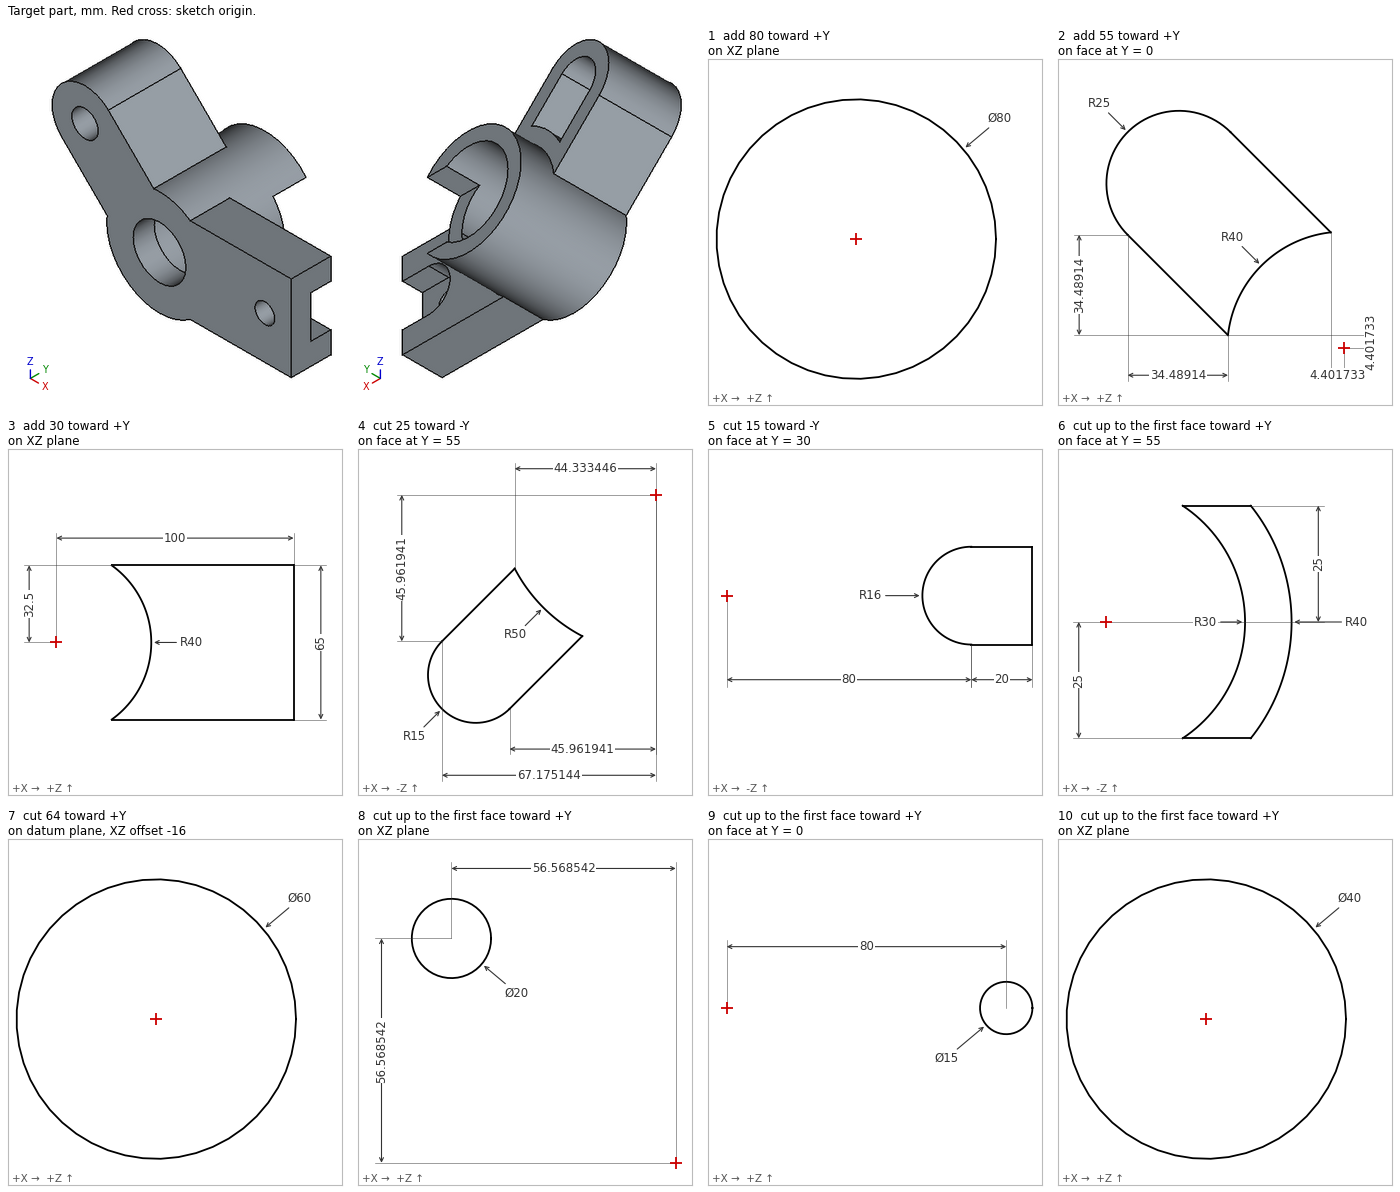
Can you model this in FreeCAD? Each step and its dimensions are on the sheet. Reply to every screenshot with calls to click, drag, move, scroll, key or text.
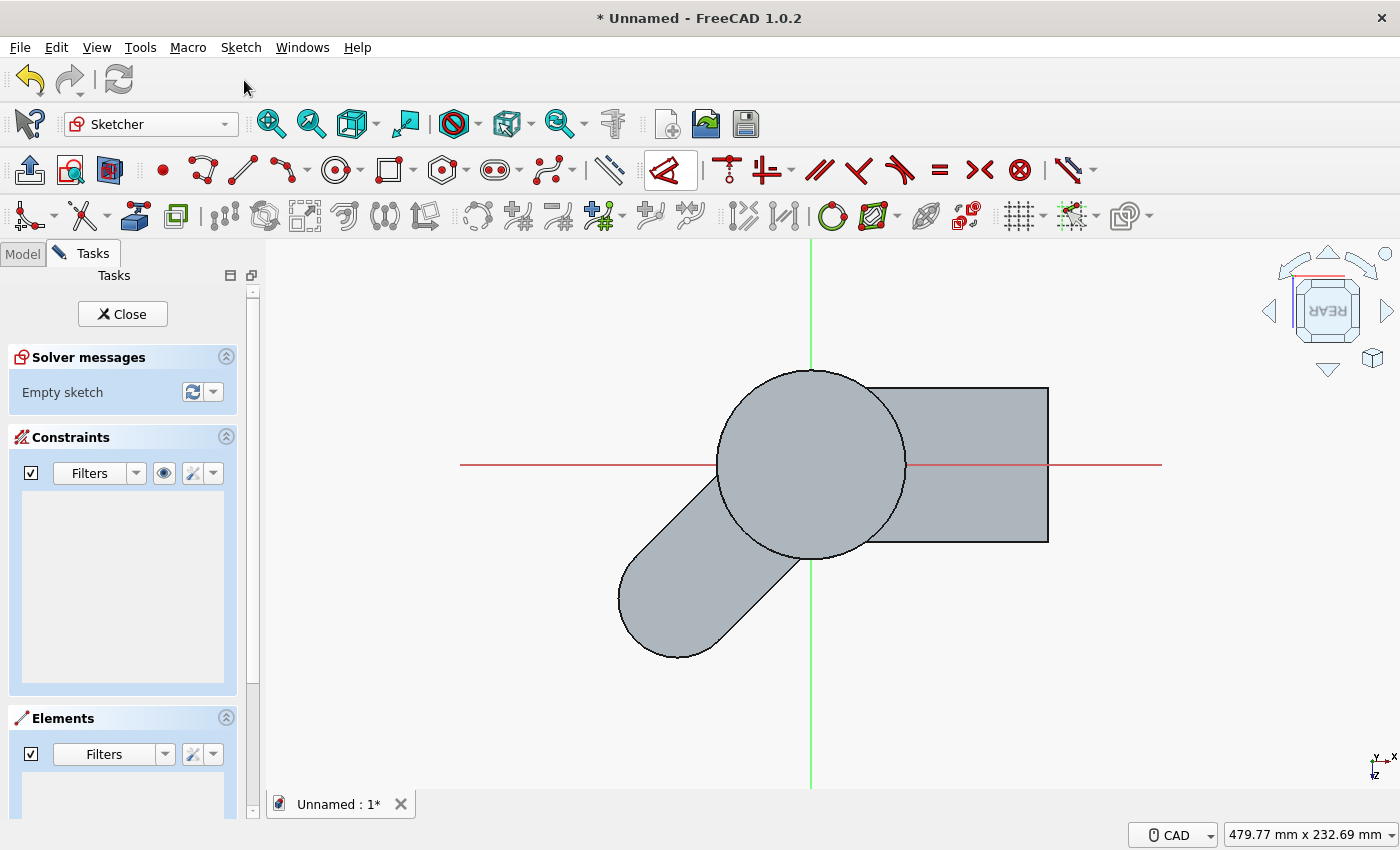
scroll(705, 569, up, 4)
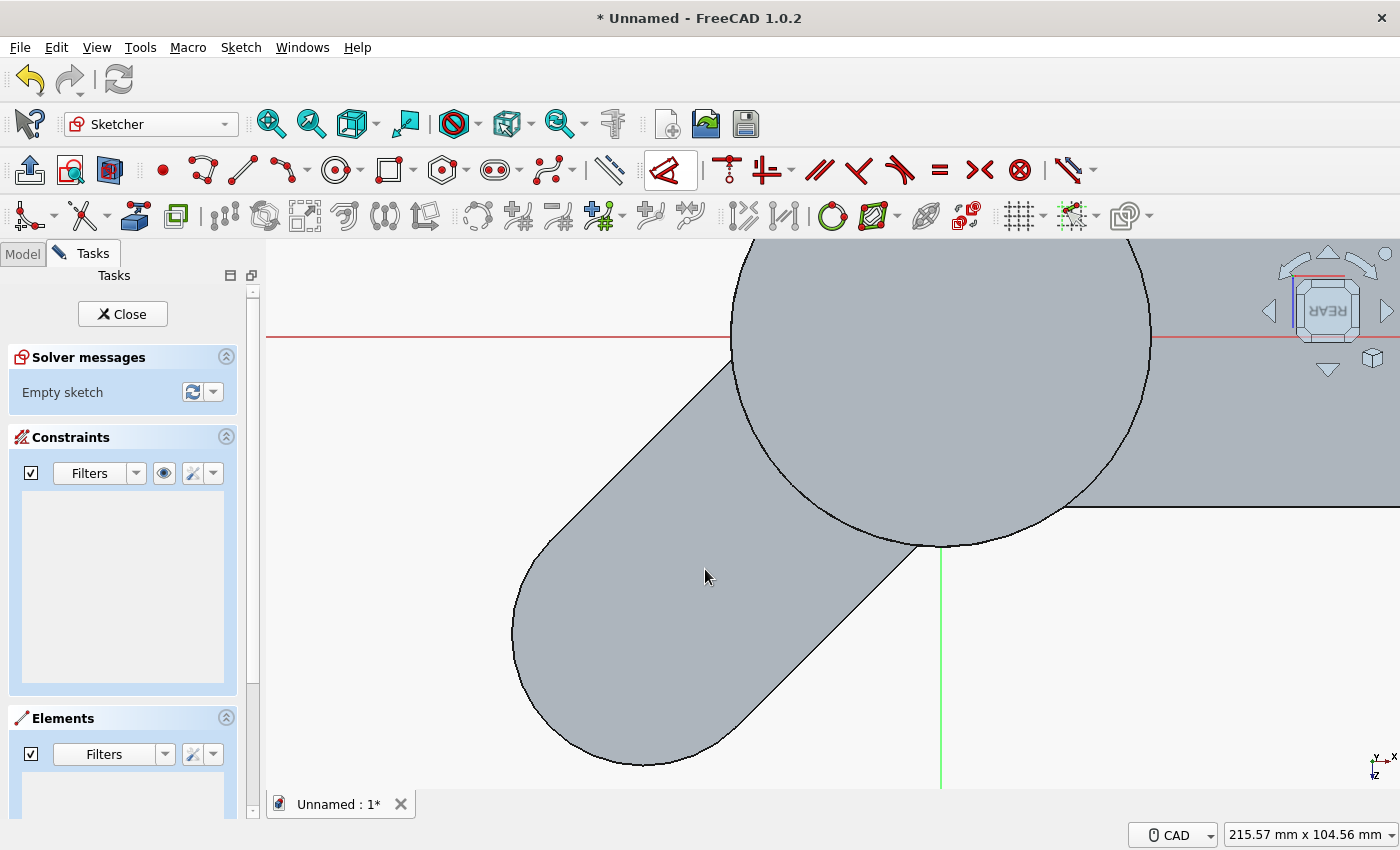
click(244, 170)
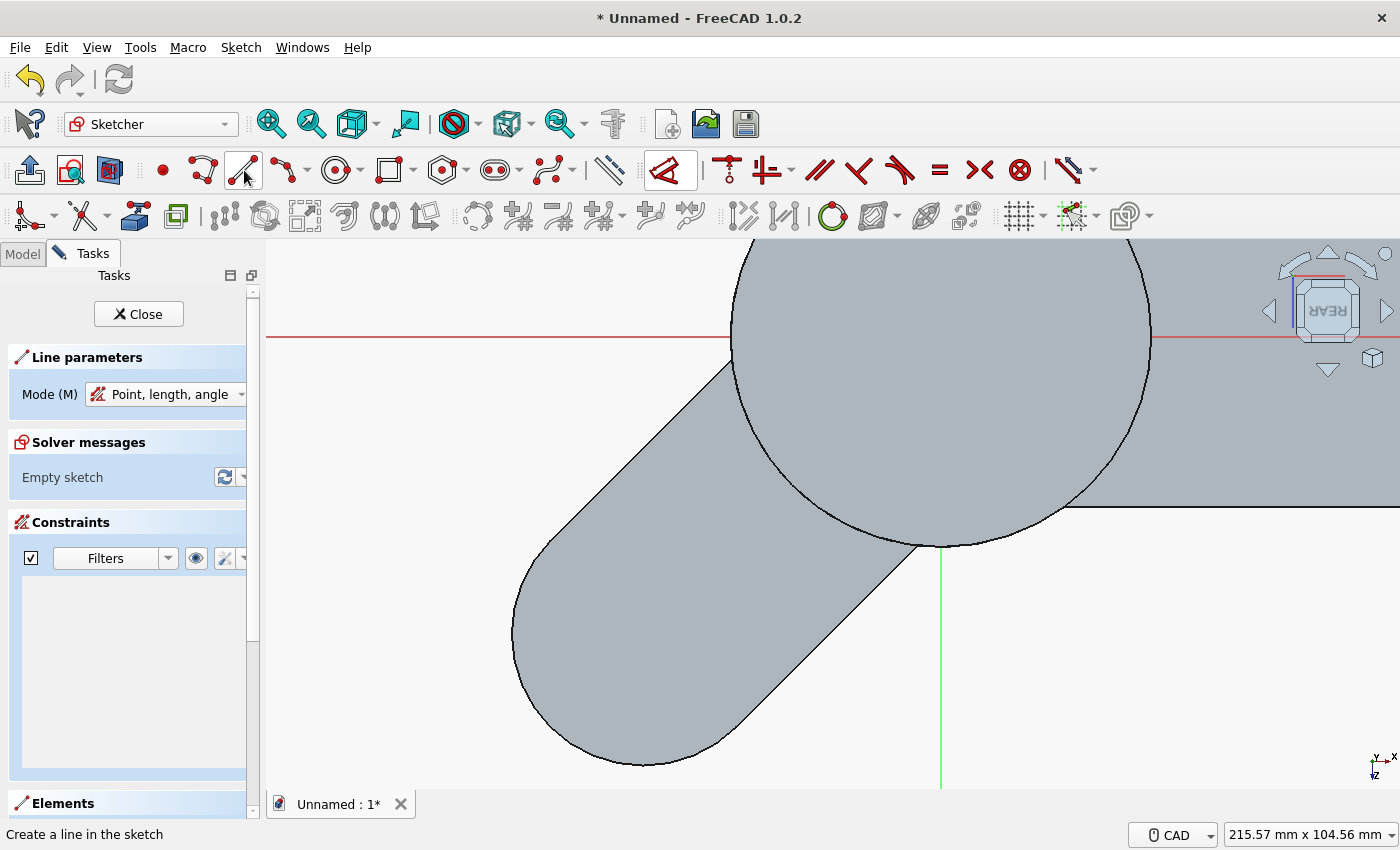
click(708, 458)
click(588, 578)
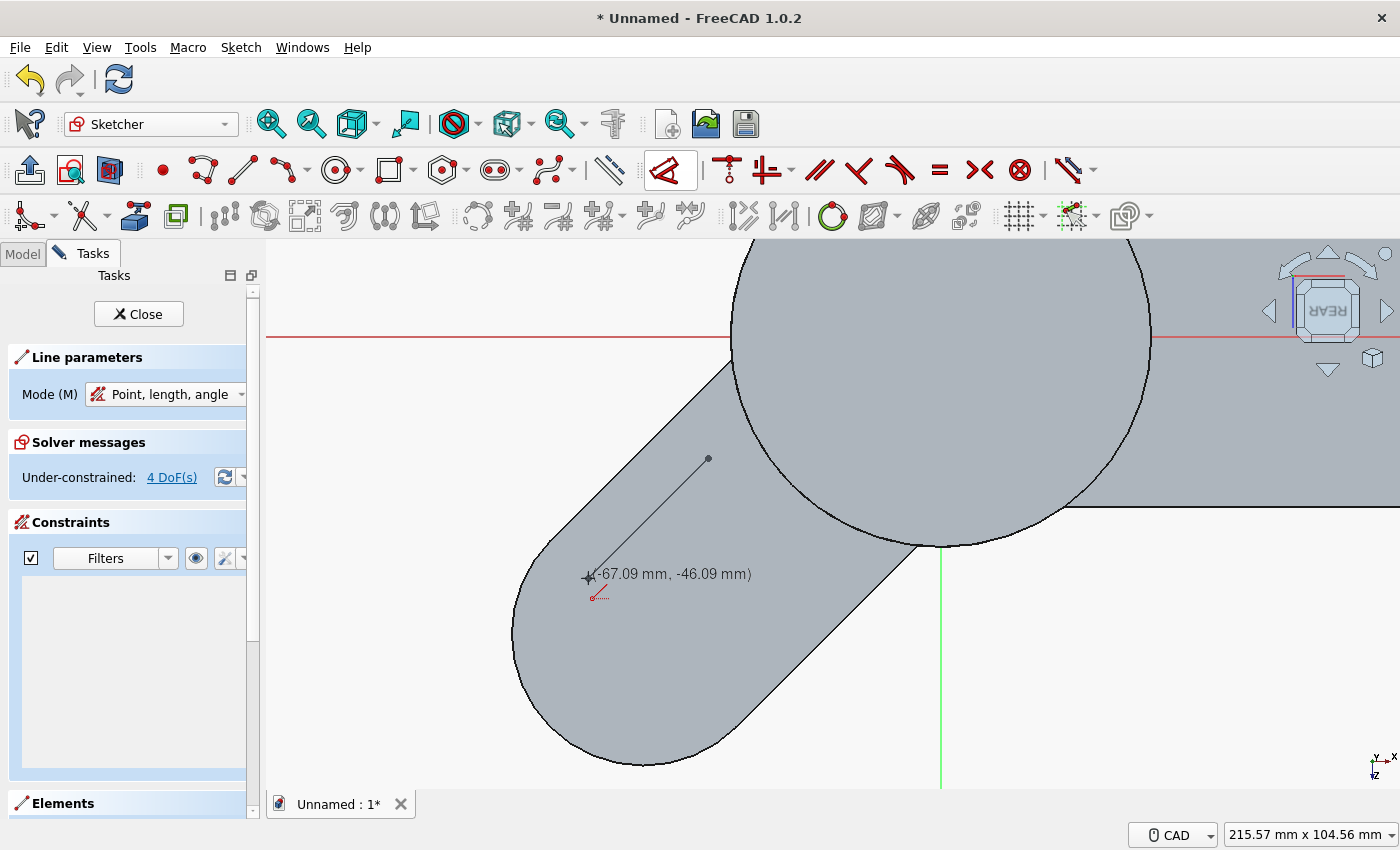
click(699, 690)
click(819, 570)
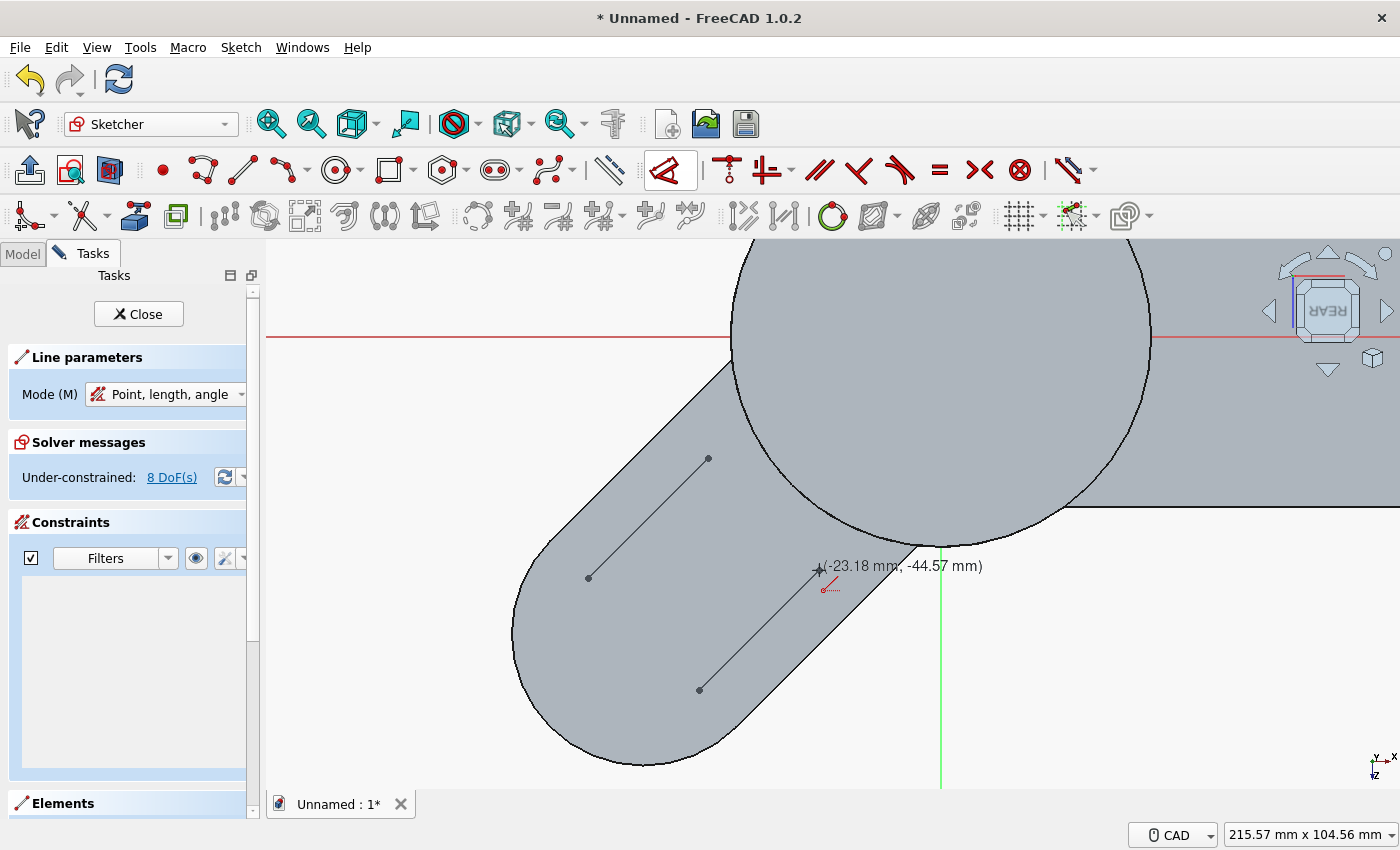
click(284, 170)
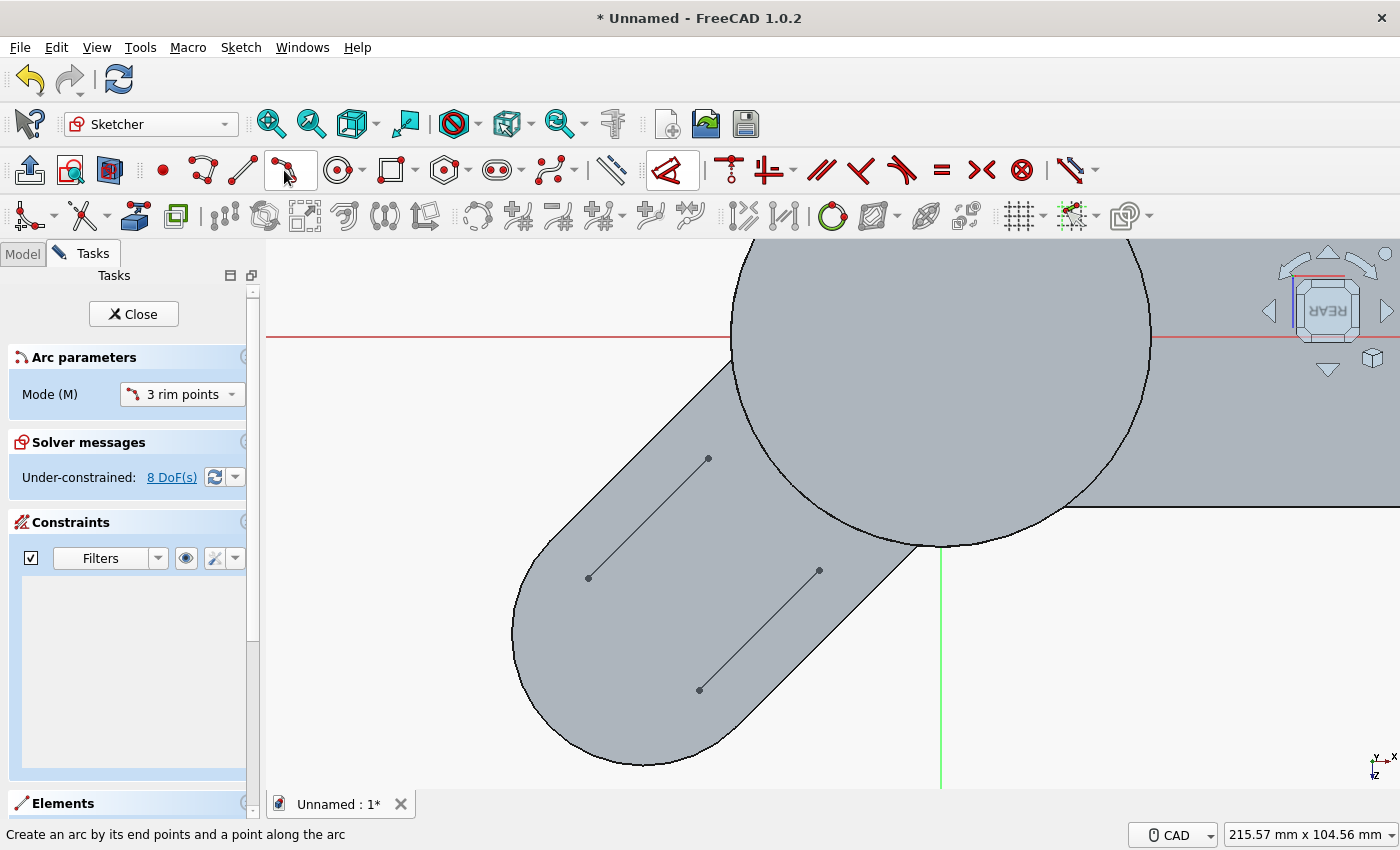
click(588, 579)
click(699, 691)
click(588, 690)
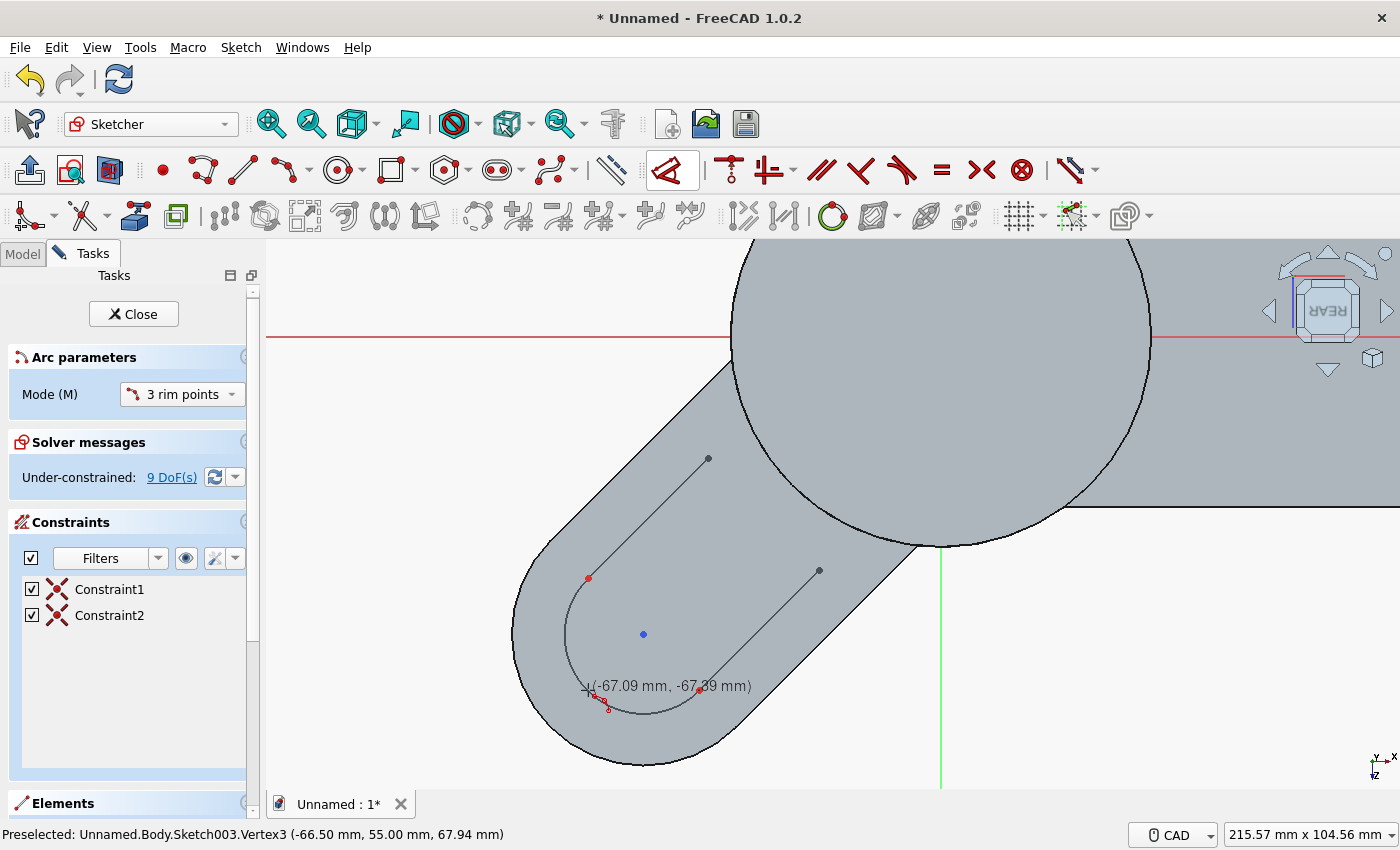
click(819, 571)
click(708, 459)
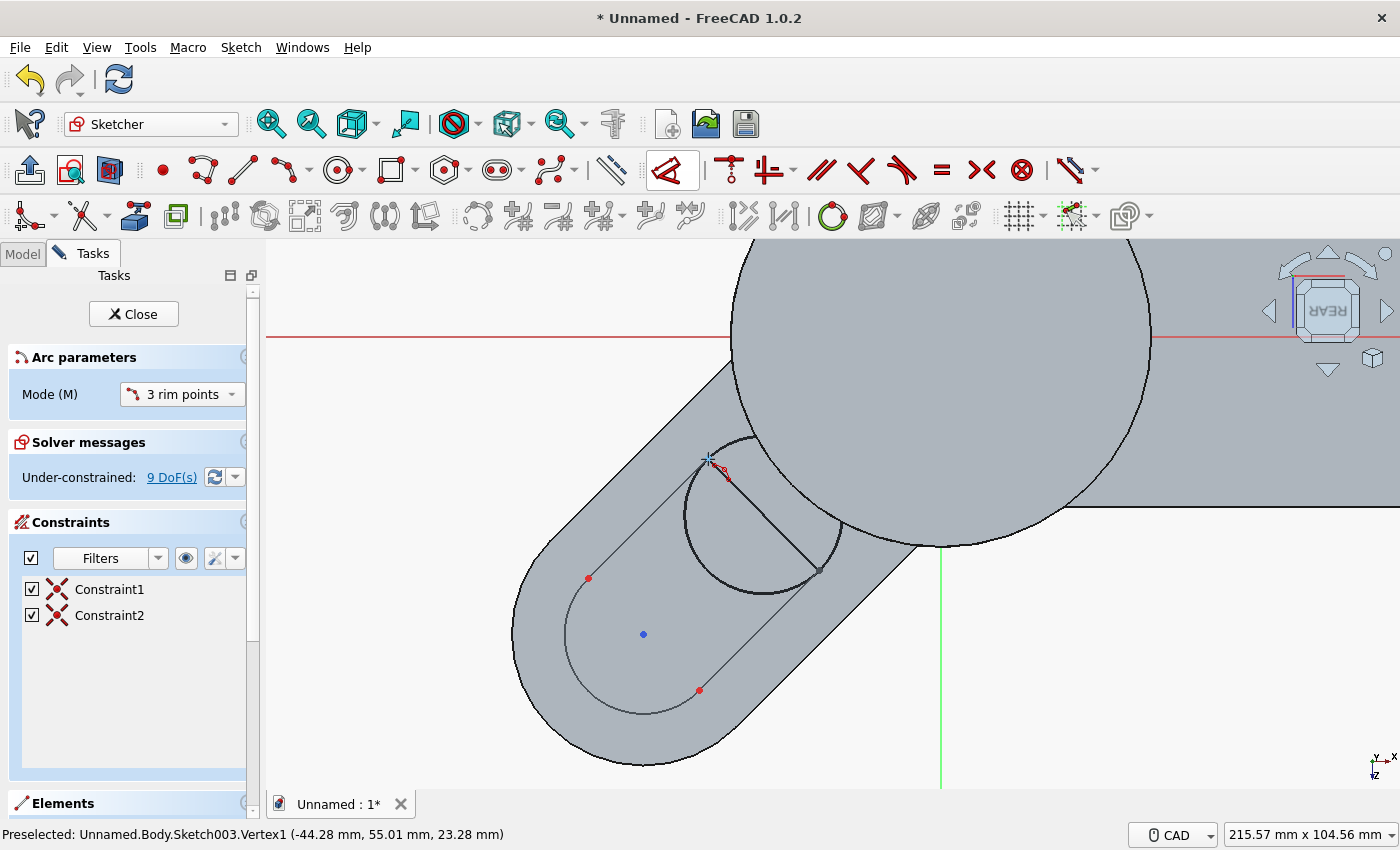
scroll(755, 523, up, 2)